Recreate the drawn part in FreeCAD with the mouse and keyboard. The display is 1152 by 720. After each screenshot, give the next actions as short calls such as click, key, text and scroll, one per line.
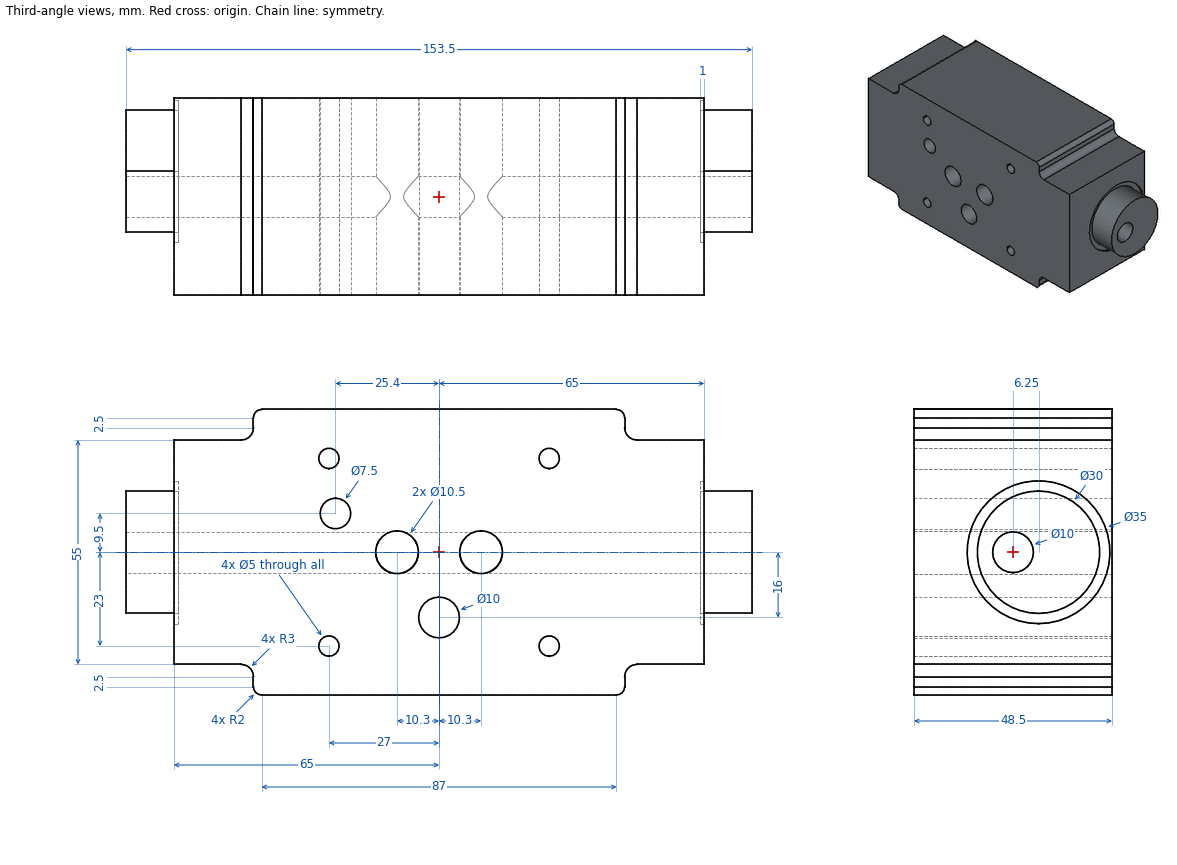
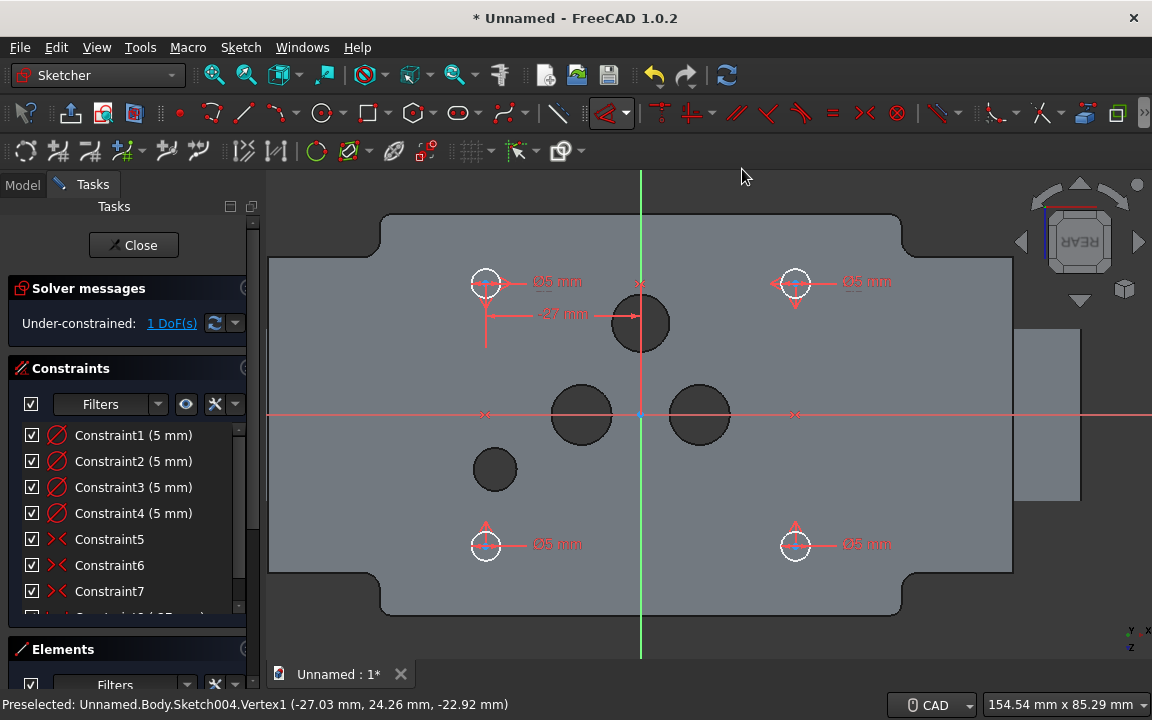
click(486, 284)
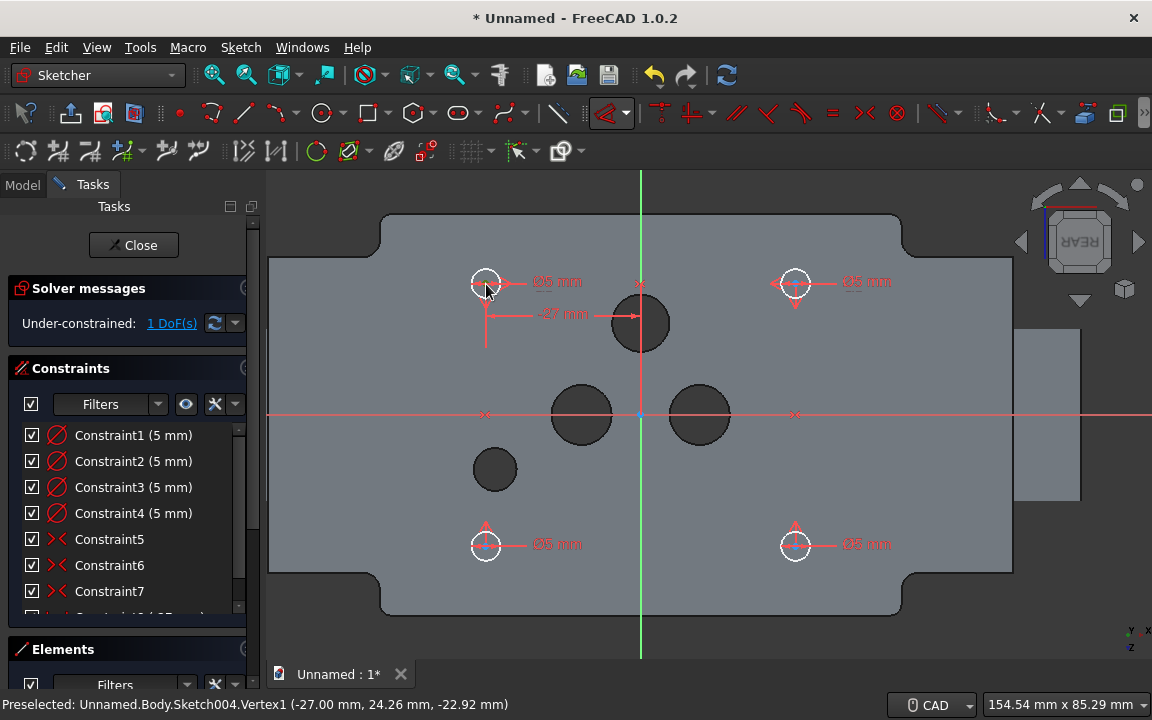
click(628, 114)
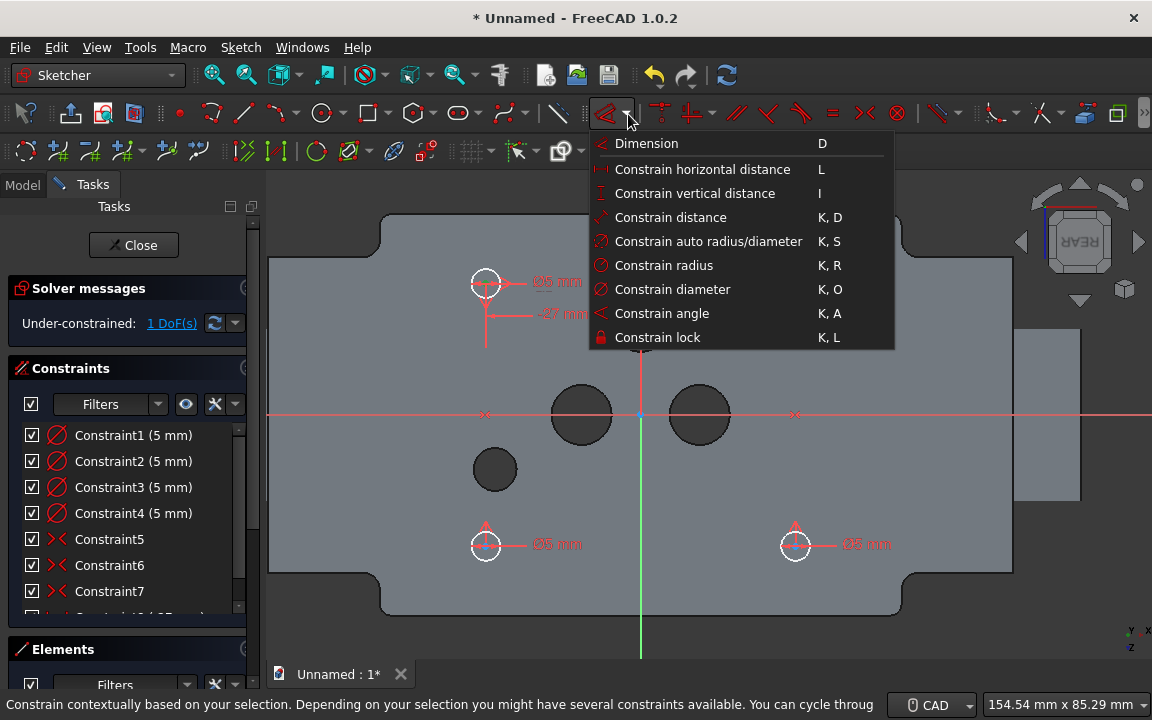
click(742, 193)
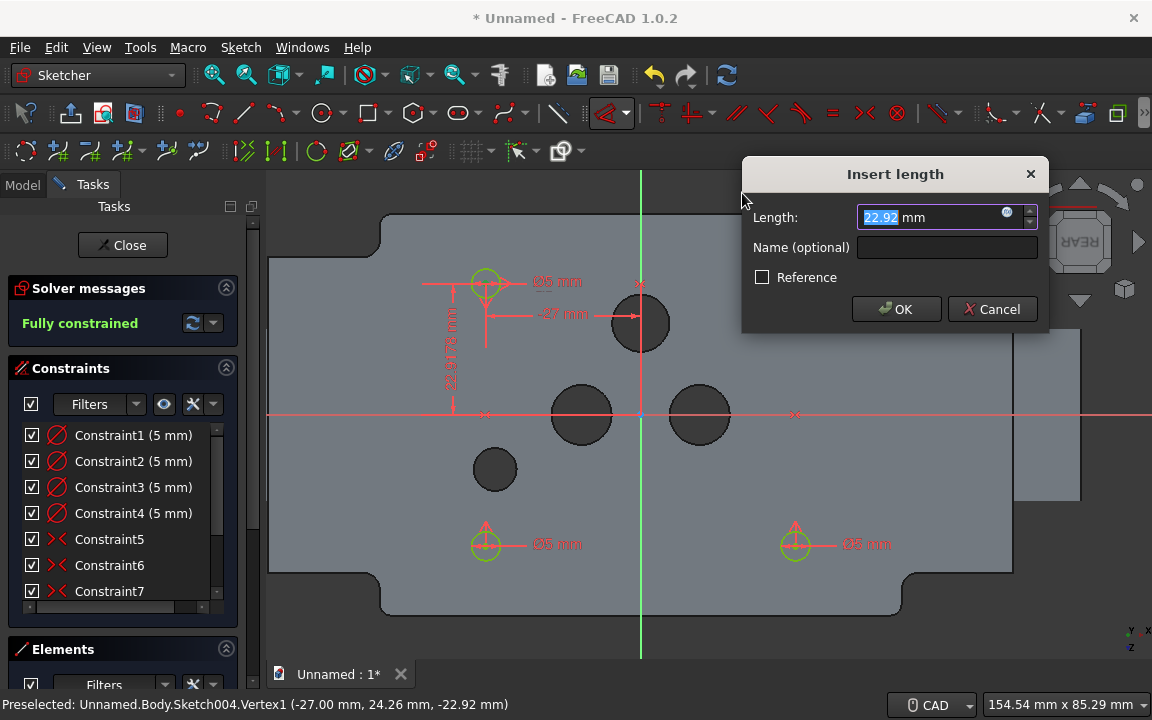
text(23)
key(Return)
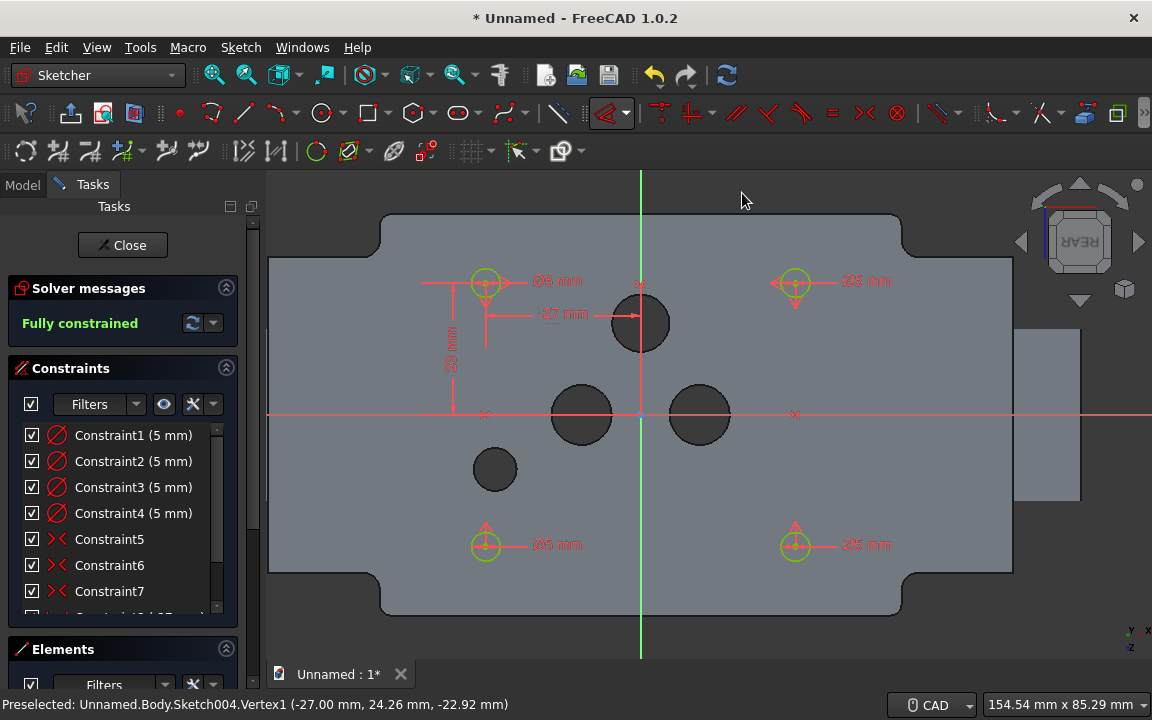
click(123, 245)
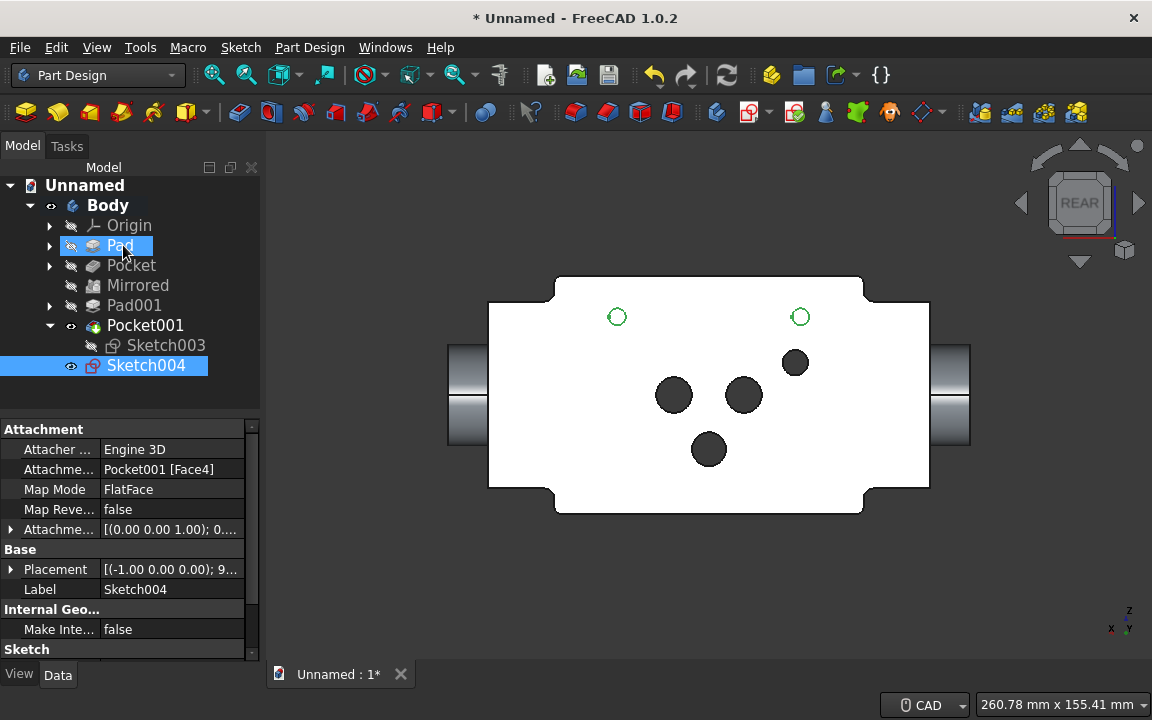
click(272, 112)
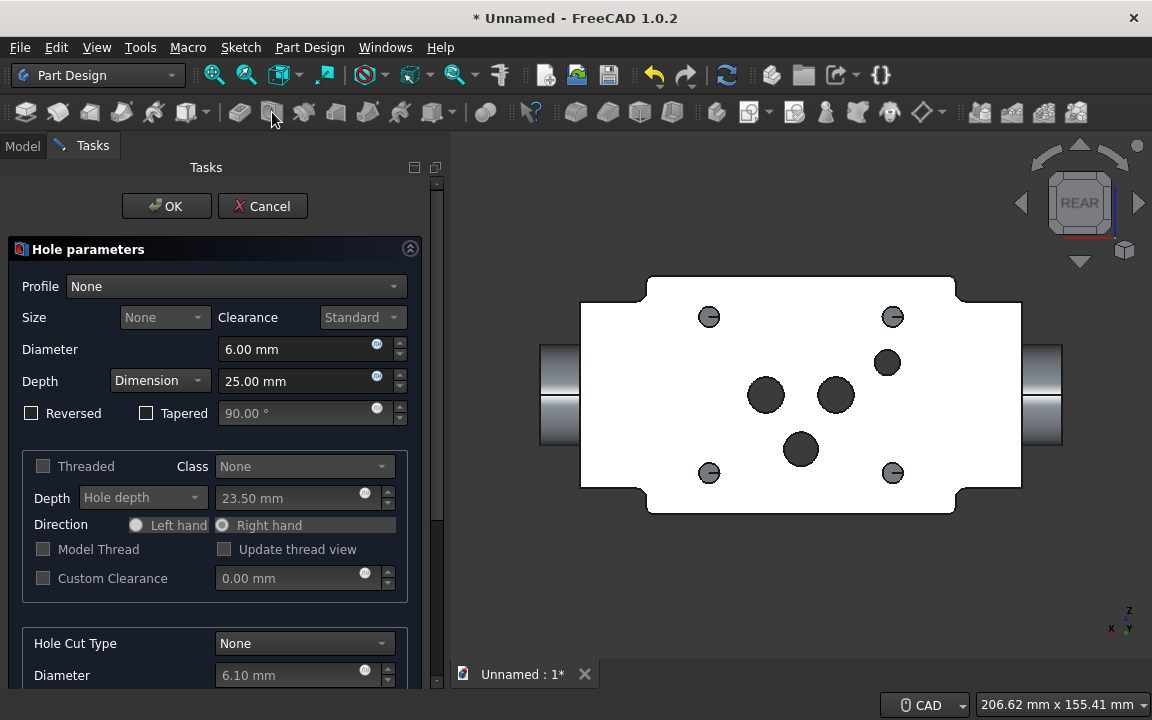
triple_click(305, 349)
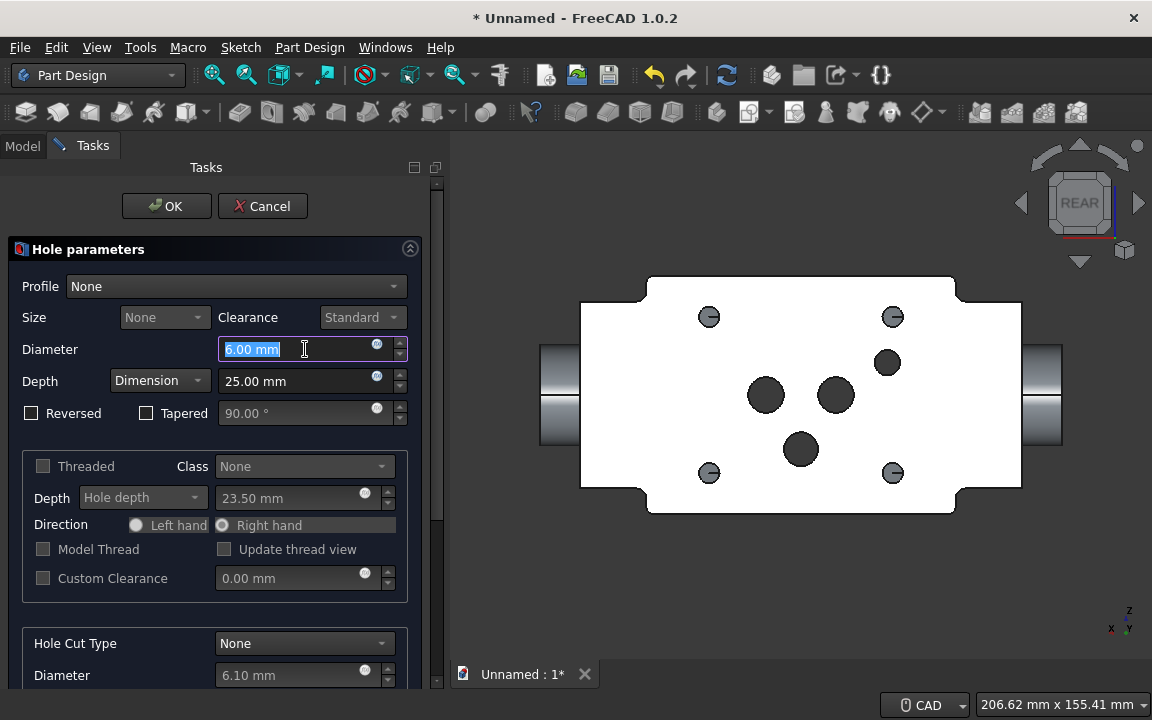
text(5)
key(Tab)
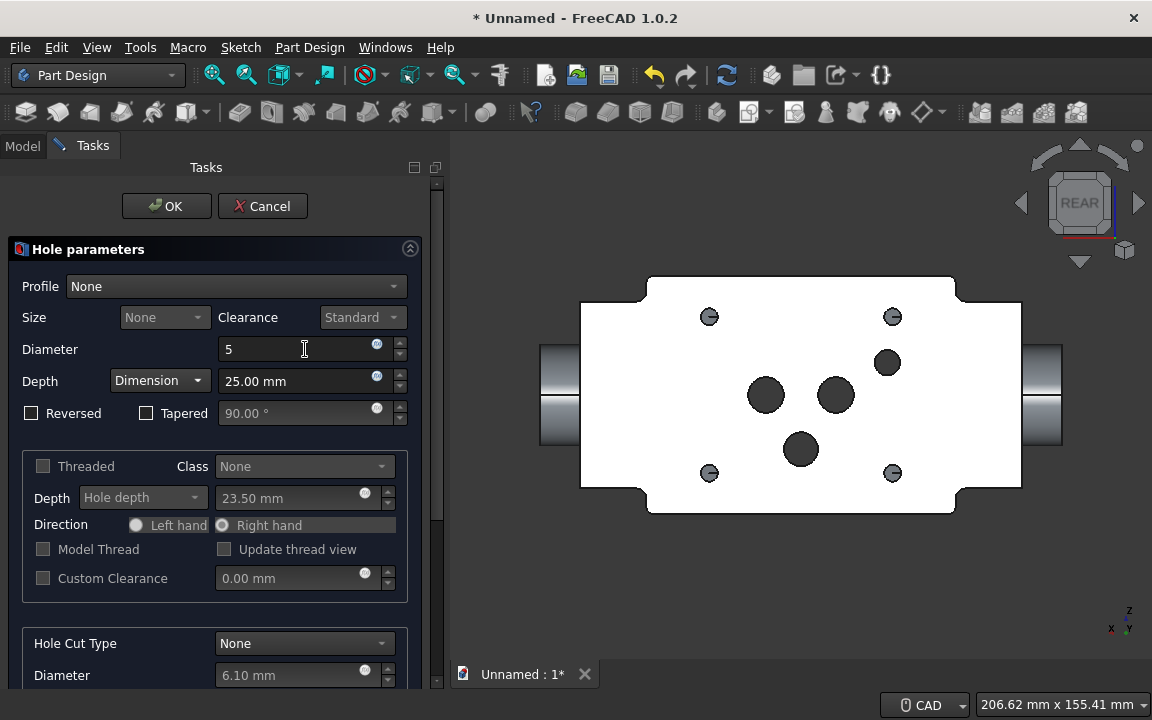
click(161, 380)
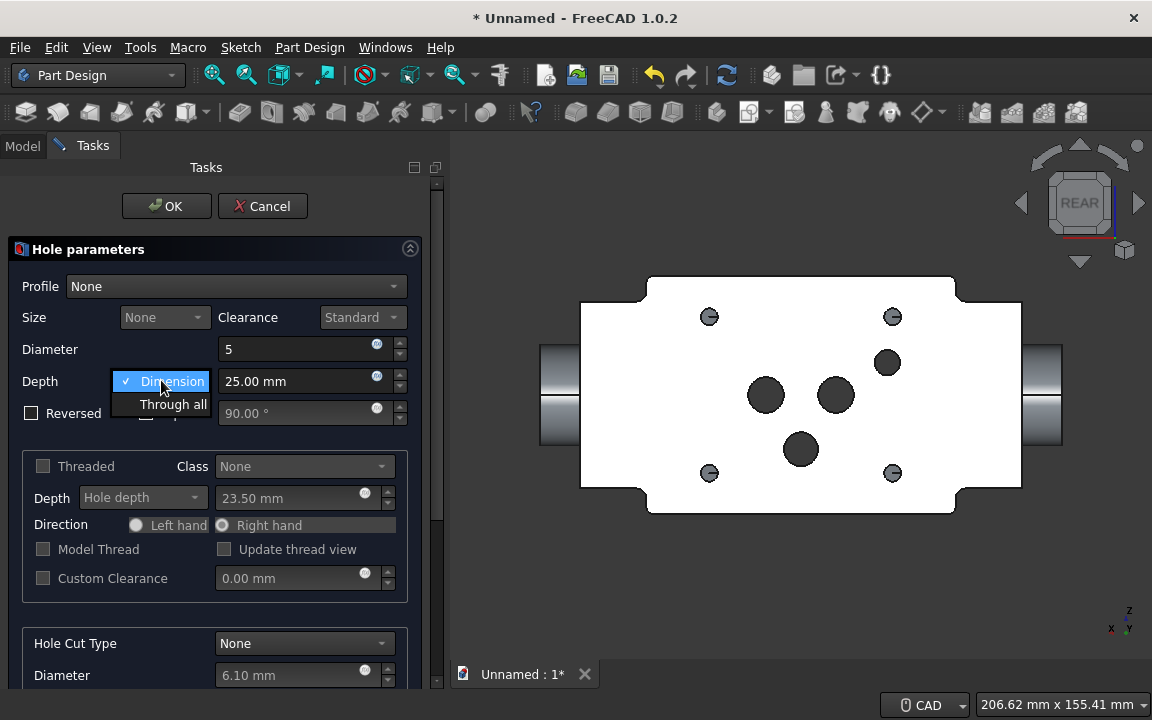
click(160, 404)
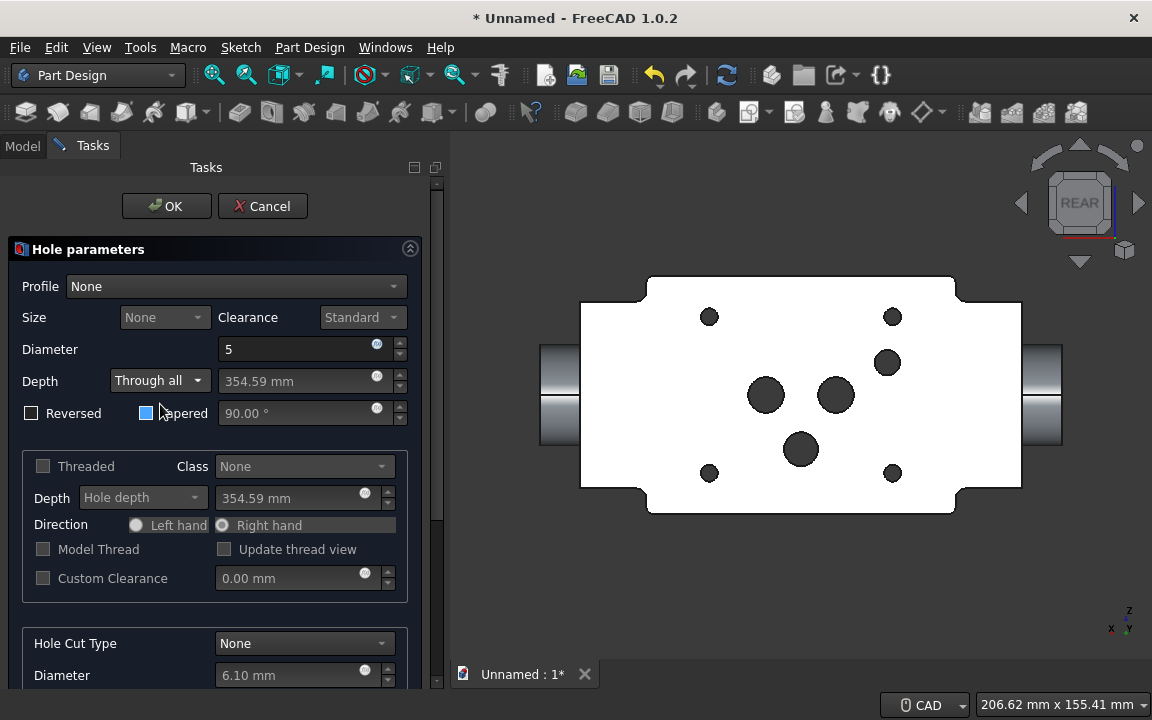
click(167, 206)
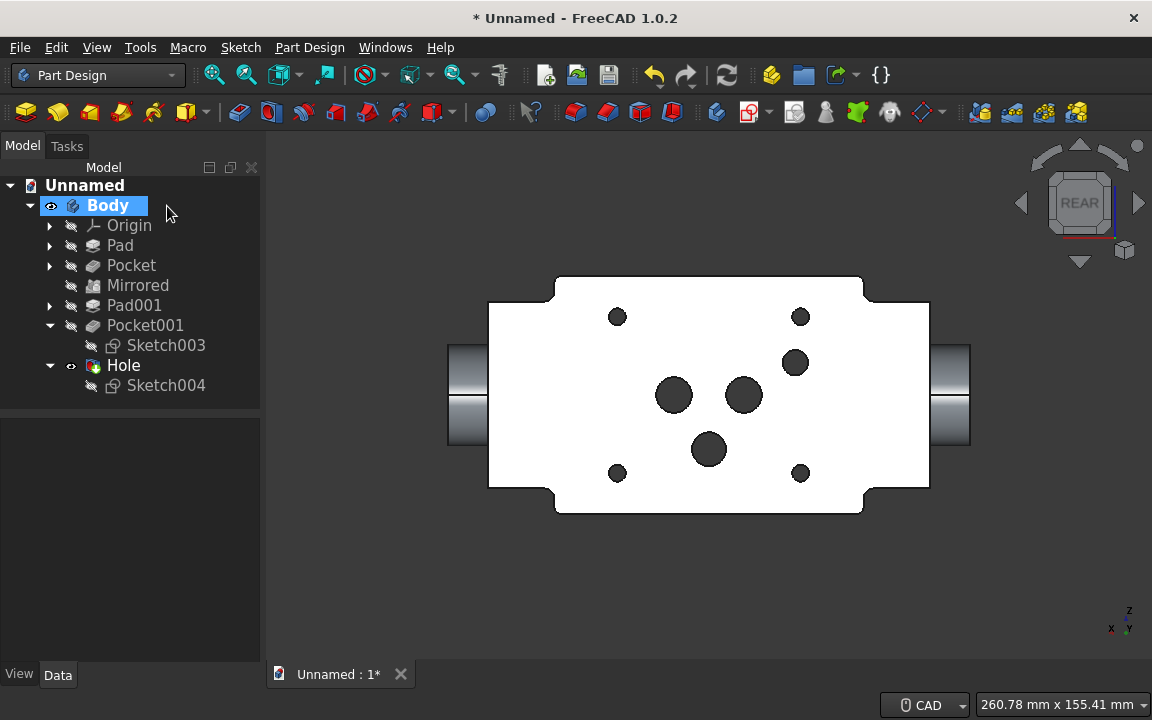
key(0)